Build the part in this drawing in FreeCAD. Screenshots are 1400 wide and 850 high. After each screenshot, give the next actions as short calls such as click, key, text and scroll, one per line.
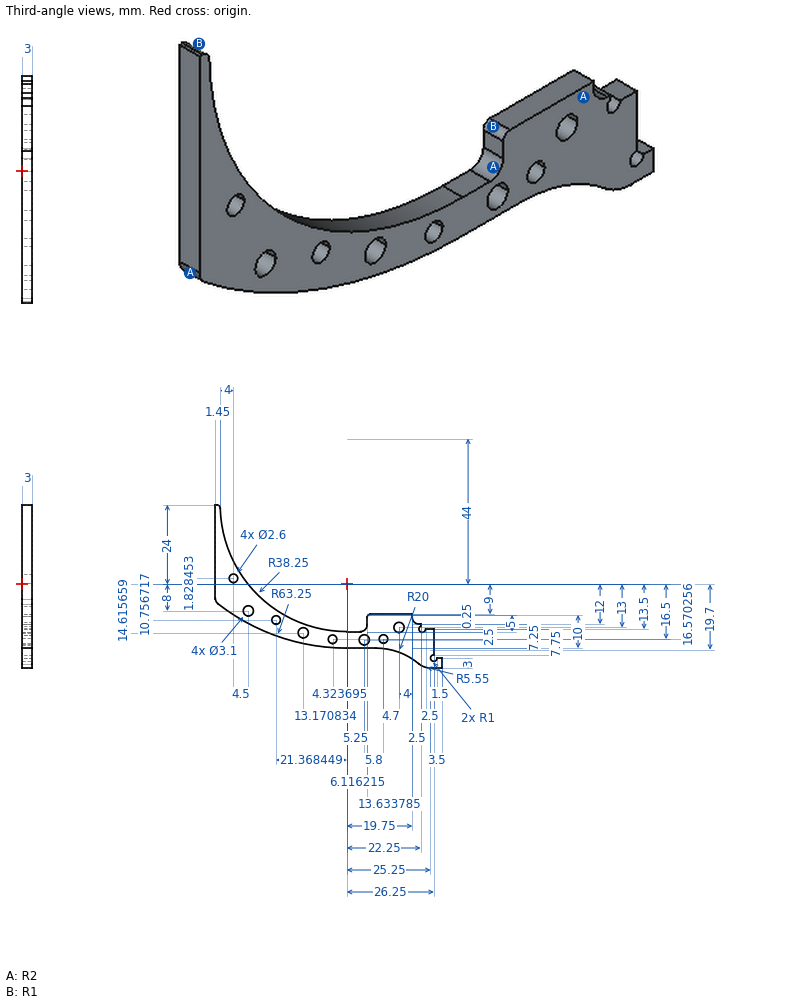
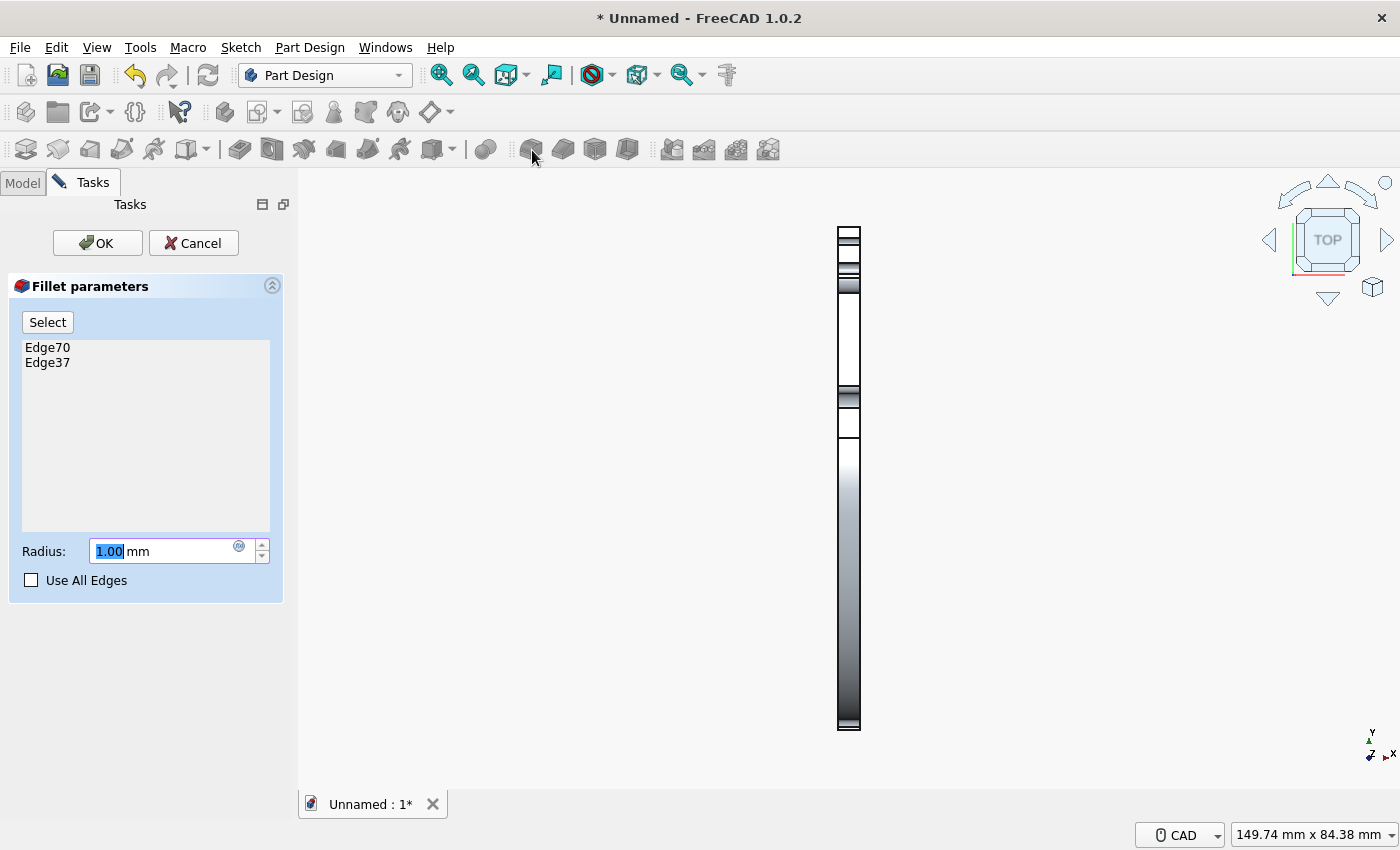
text(1)
key(Tab)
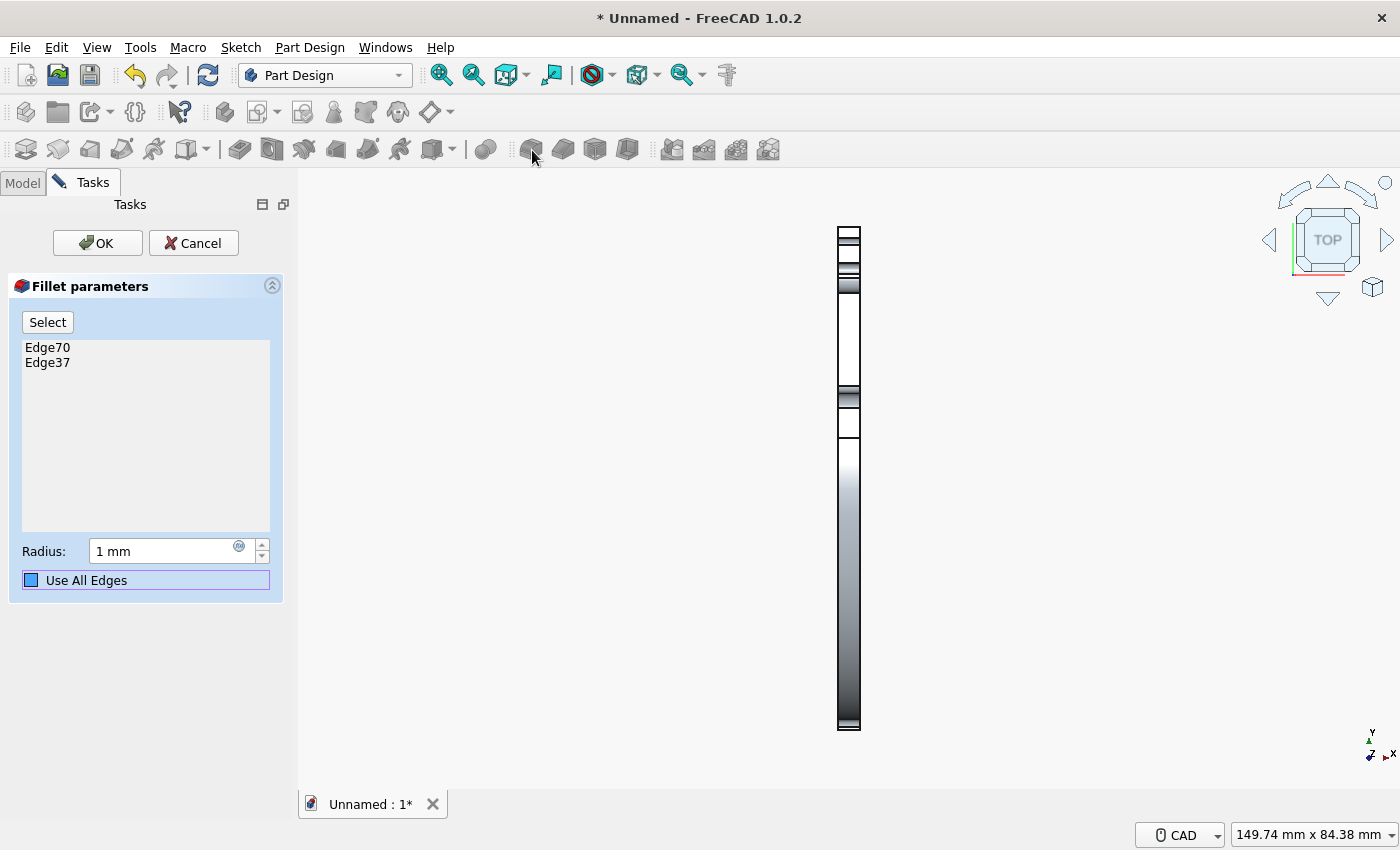
click(98, 243)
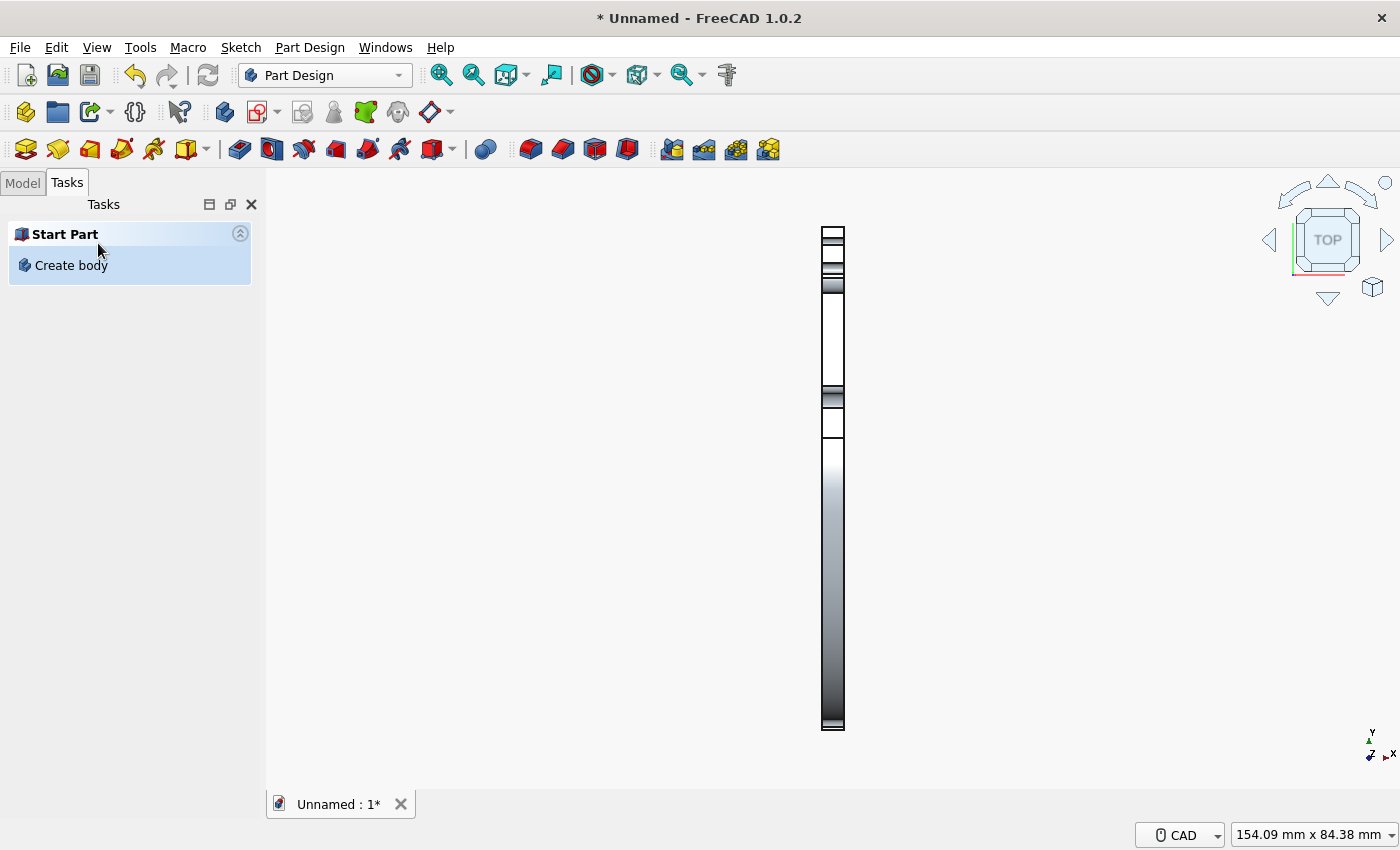
key(0)